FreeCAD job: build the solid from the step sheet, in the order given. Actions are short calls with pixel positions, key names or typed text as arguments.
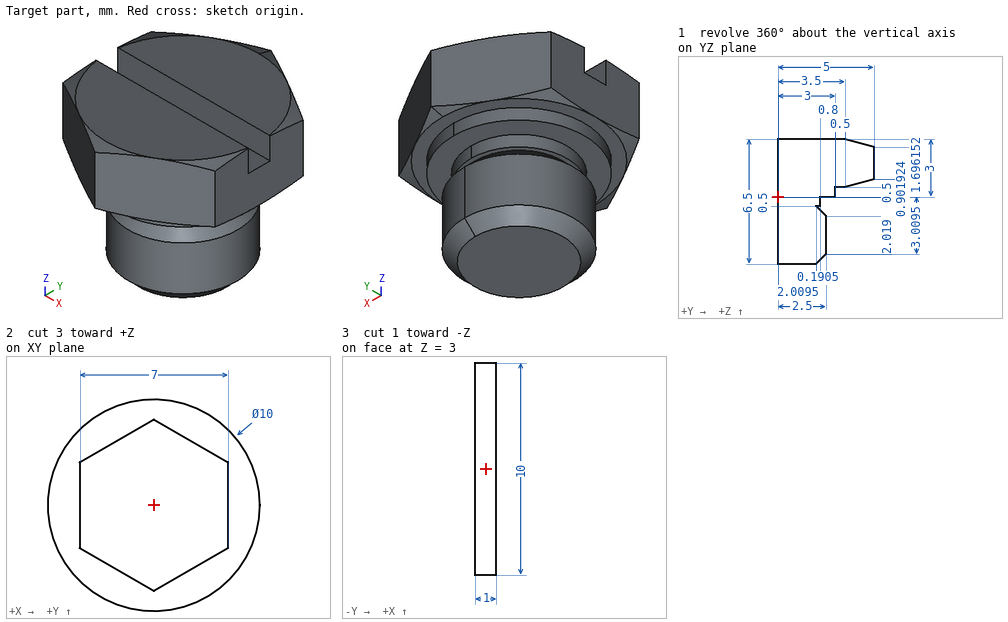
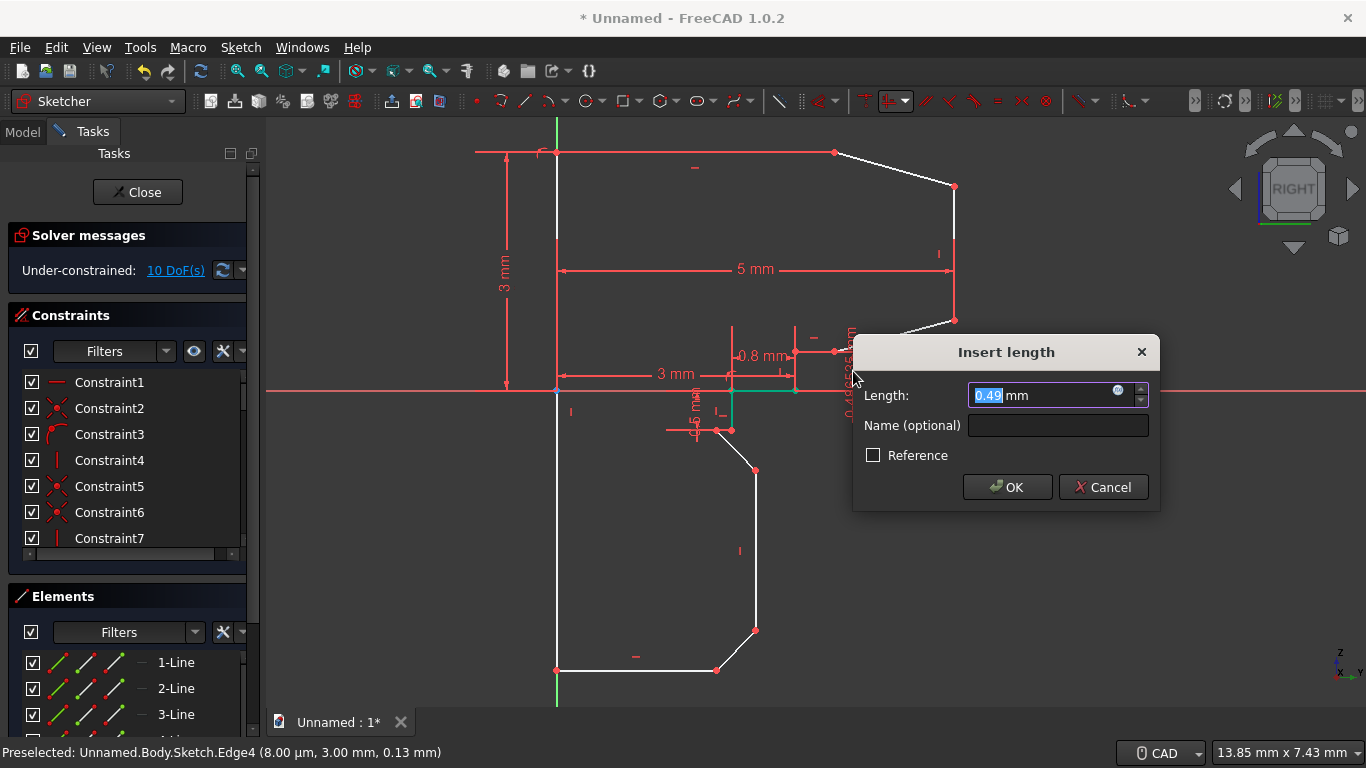
text(0.5)
key(Return)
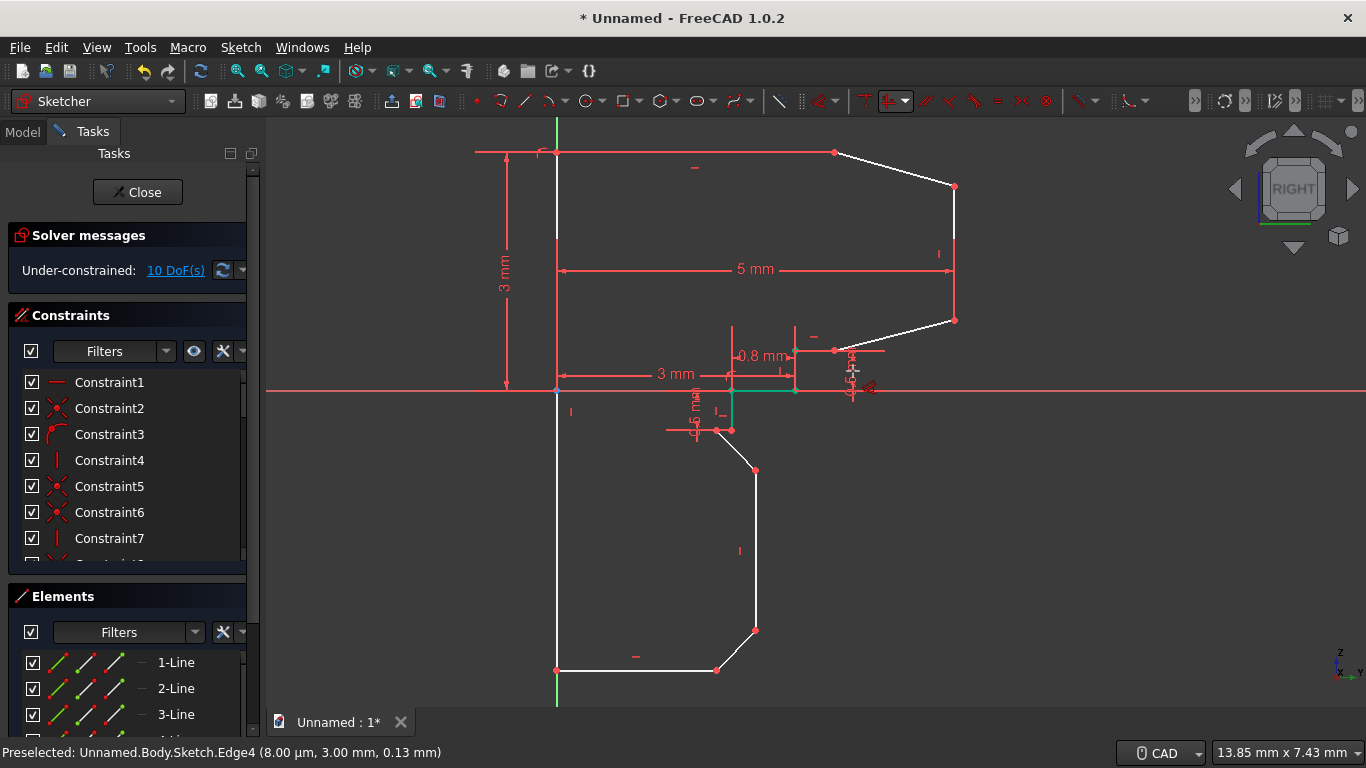
click(807, 351)
click(815, 317)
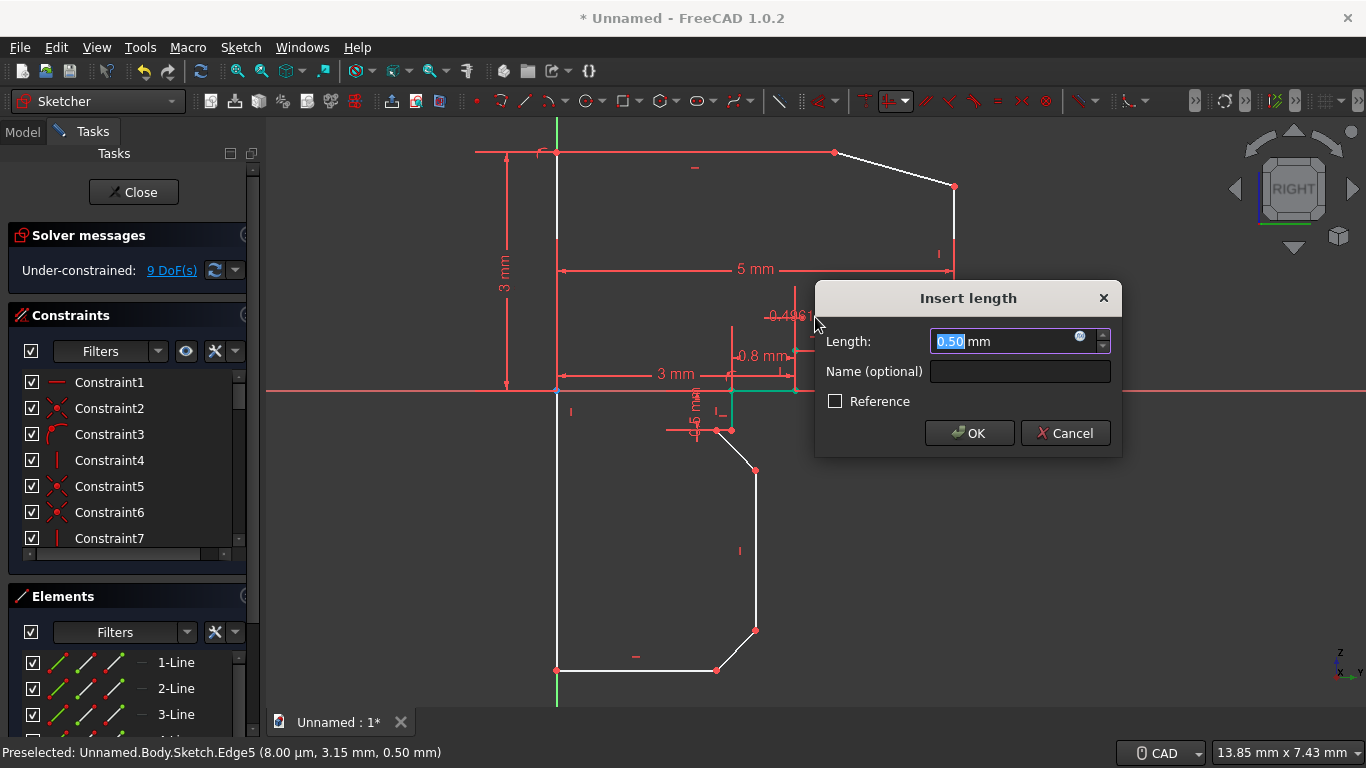
text(0.5)
key(Return)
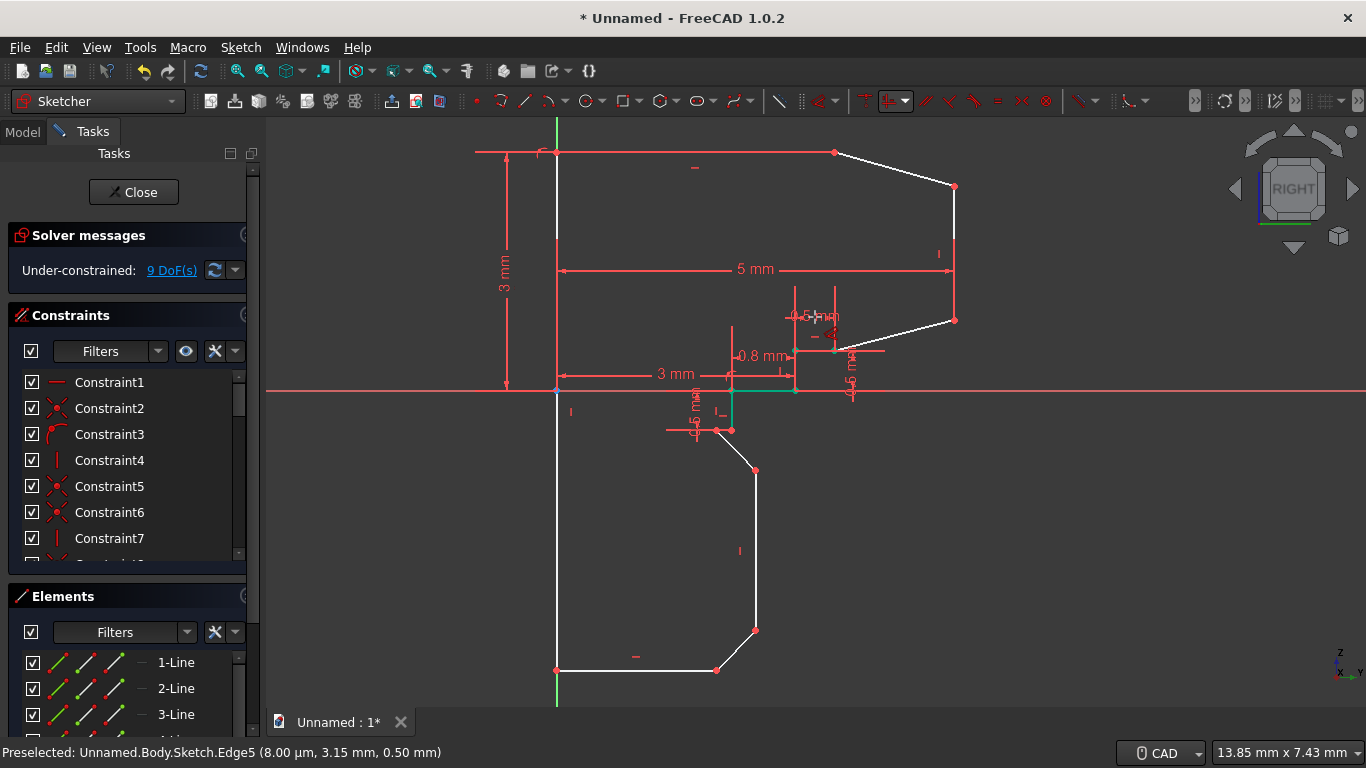
click(751, 152)
click(696, 186)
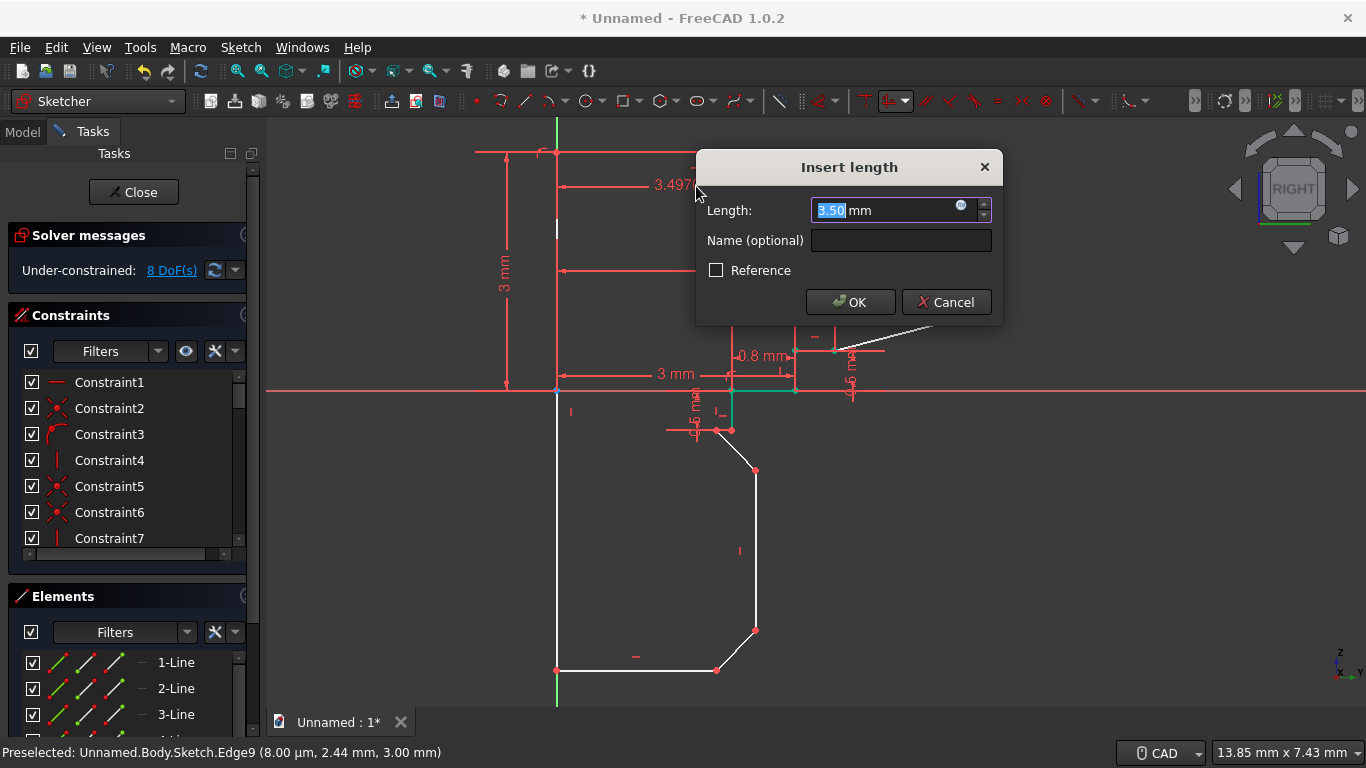
text(3.5)
key(Return)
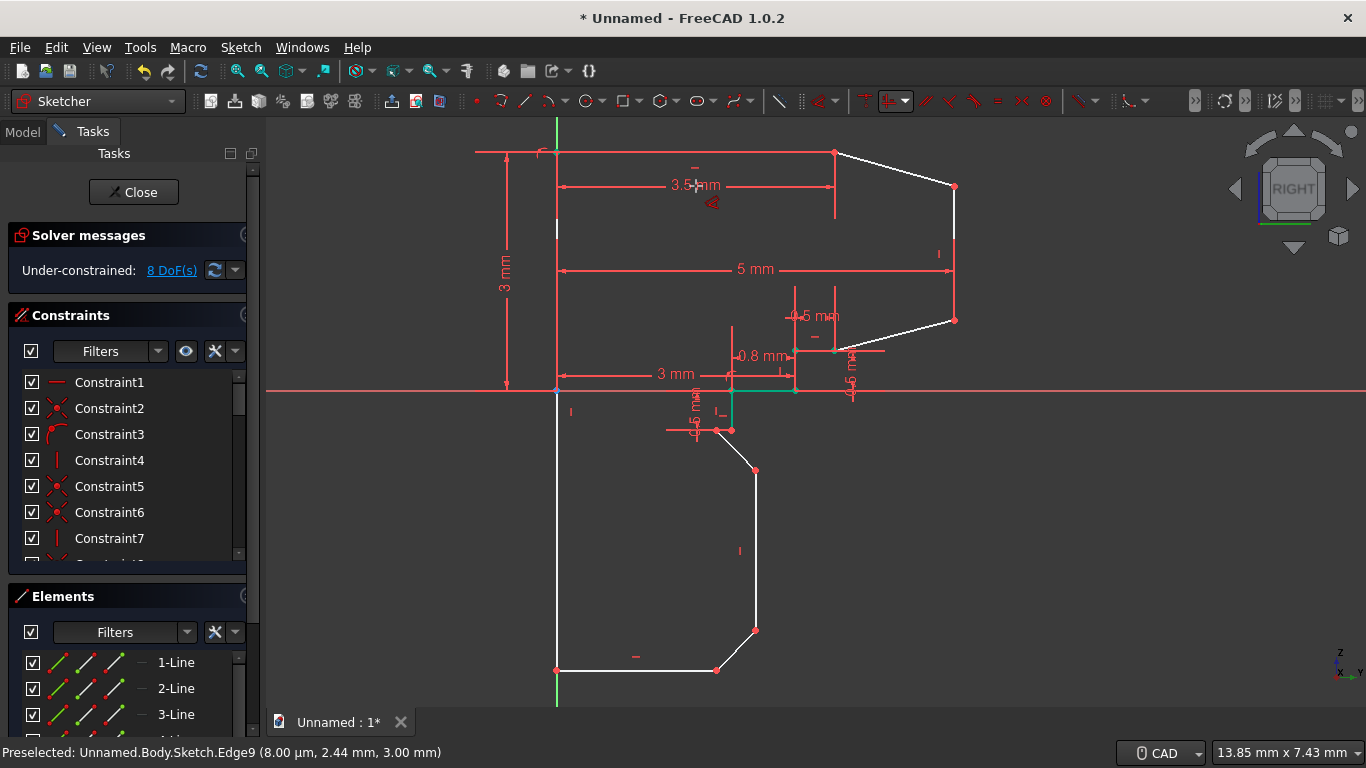
click(557, 308)
click(523, 412)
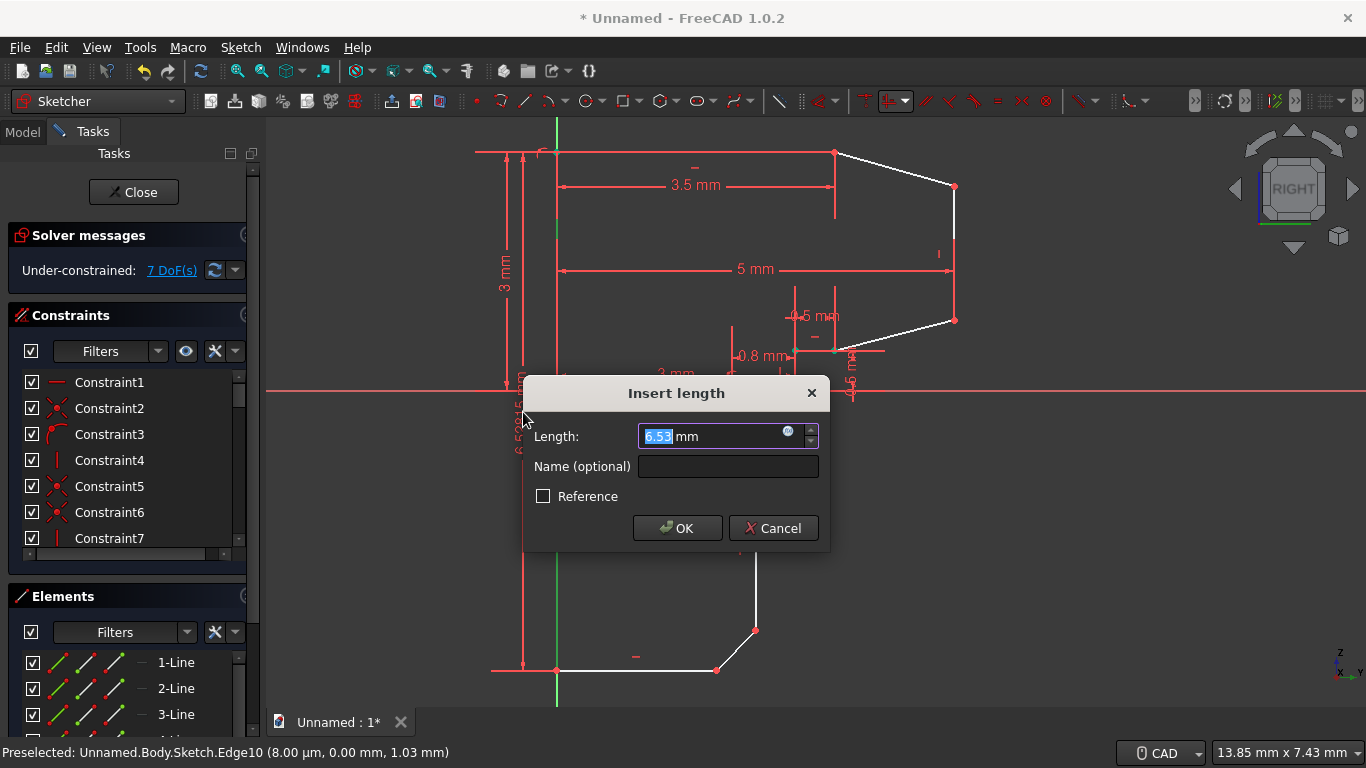
text(6.5)
key(Return)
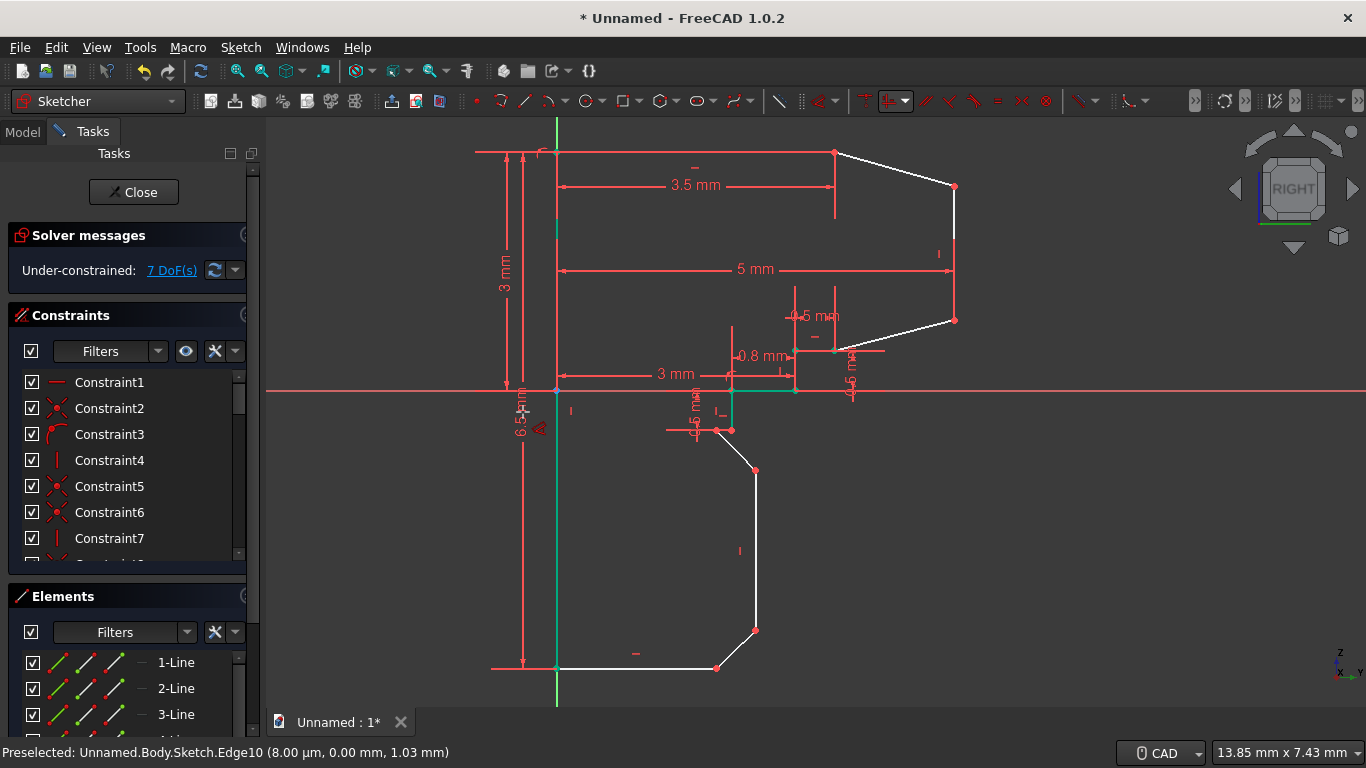
click(756, 631)
click(587, 357)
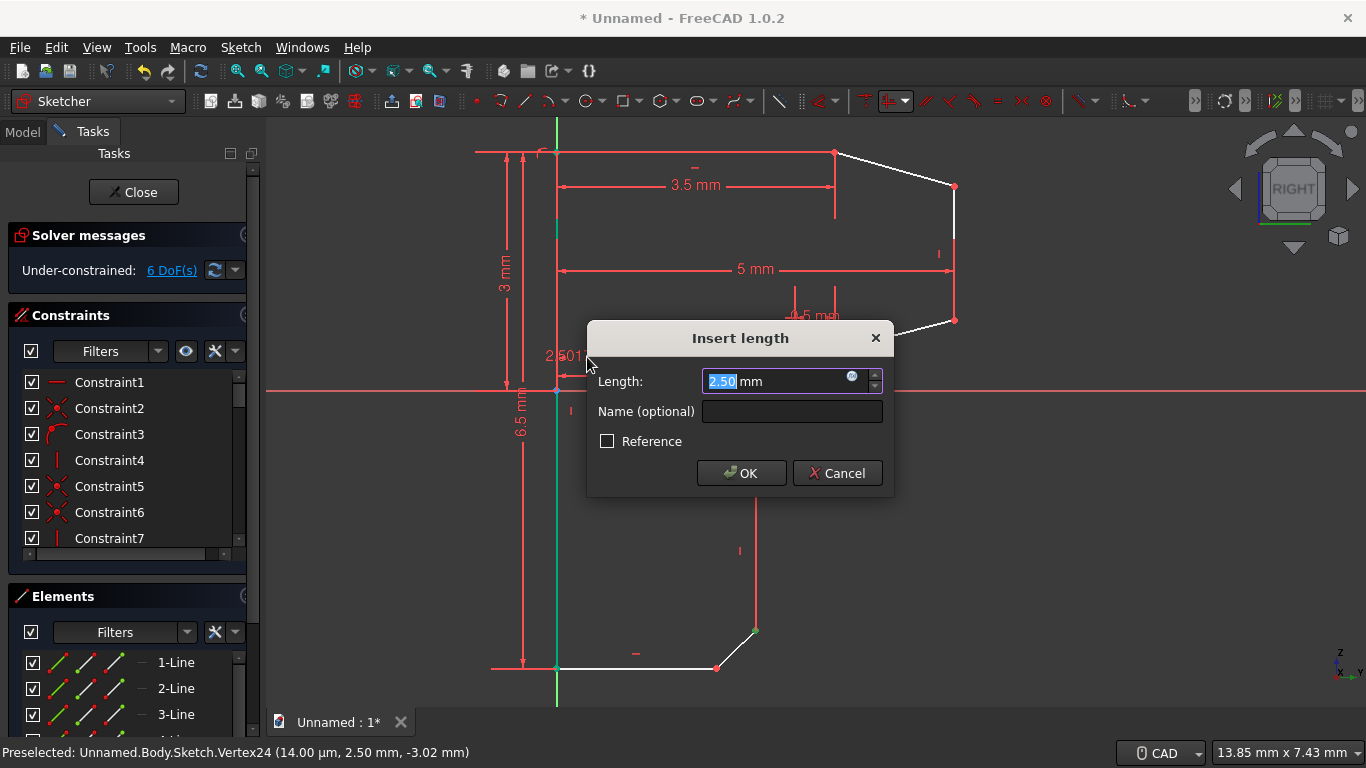
text(2.5)
key(Return)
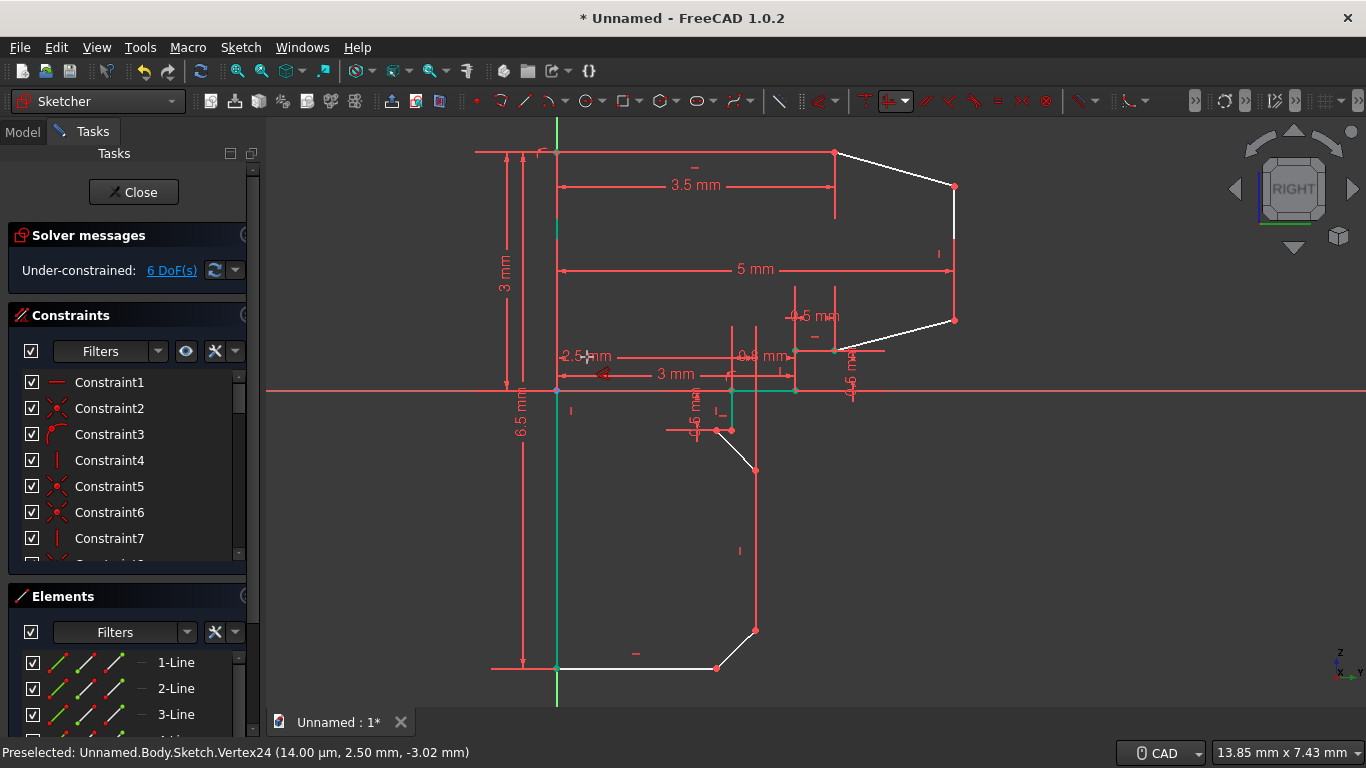
click(756, 583)
click(790, 551)